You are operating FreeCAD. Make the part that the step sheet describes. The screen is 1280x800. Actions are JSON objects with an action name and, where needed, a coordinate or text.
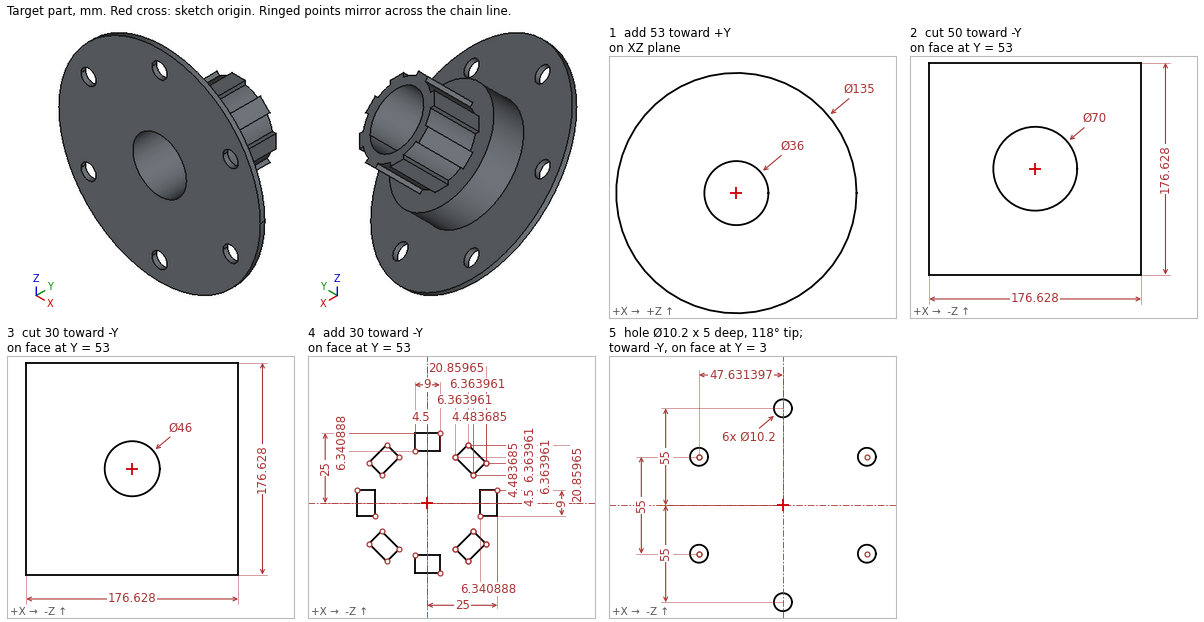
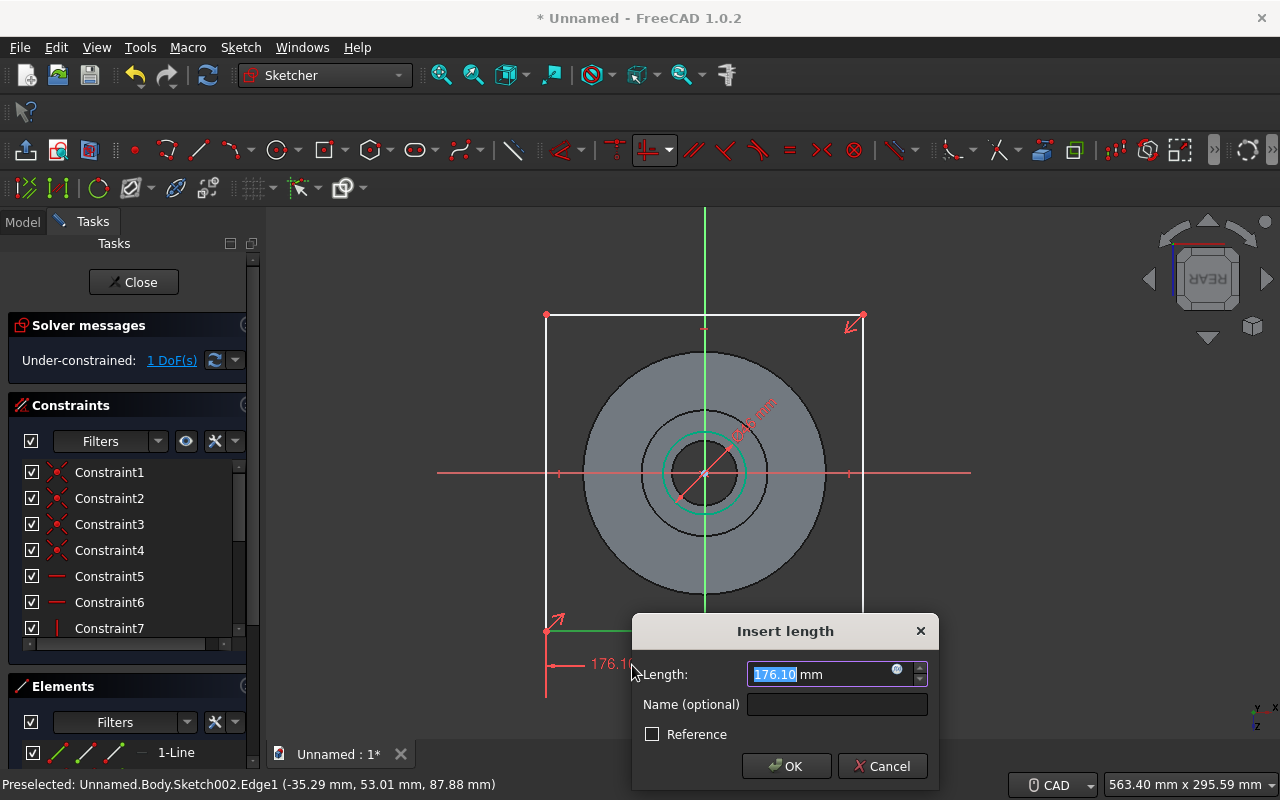
{"action": "type", "text": "176.628"}
{"action": "key", "text": "Return"}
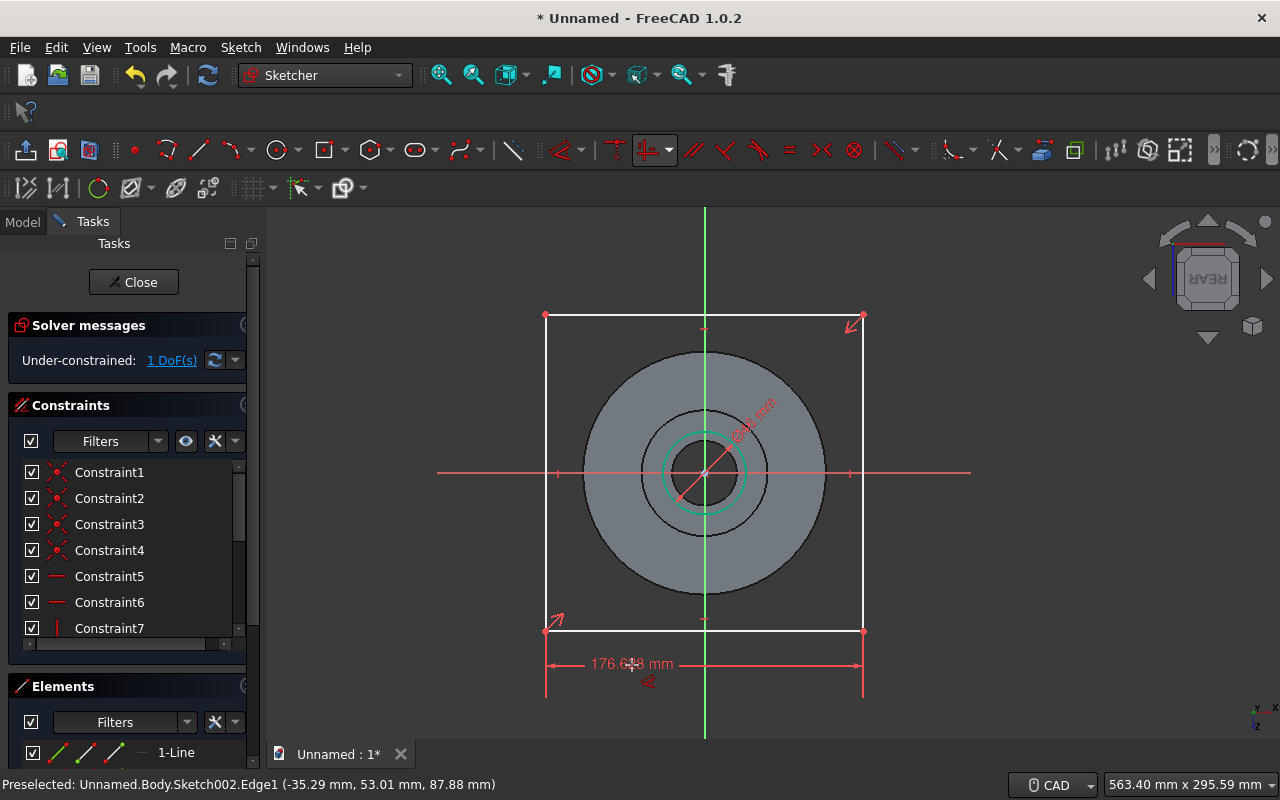
{"action": "left_click", "coordinate": [863, 536]}
{"action": "left_click", "coordinate": [897, 400]}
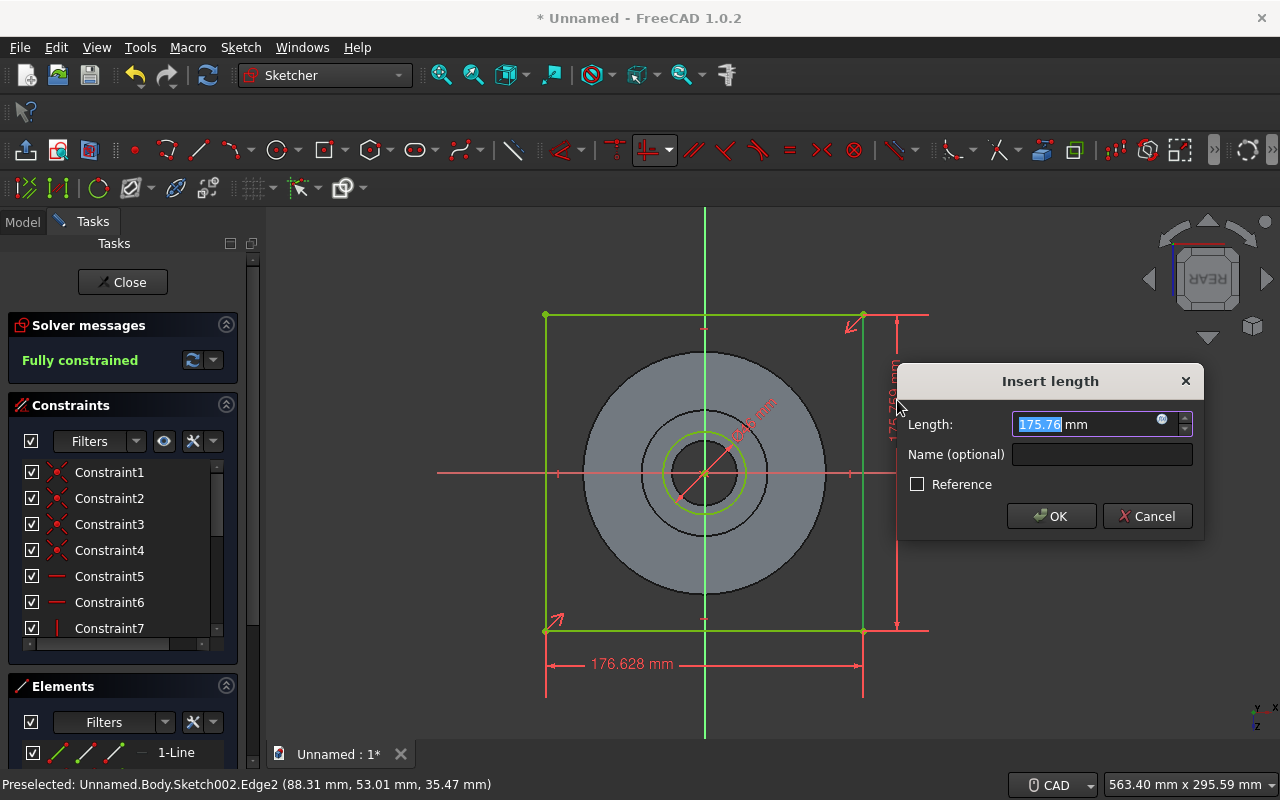
{"action": "type", "text": "176.628"}
{"action": "key", "text": "Return"}
{"action": "key", "text": "Escape"}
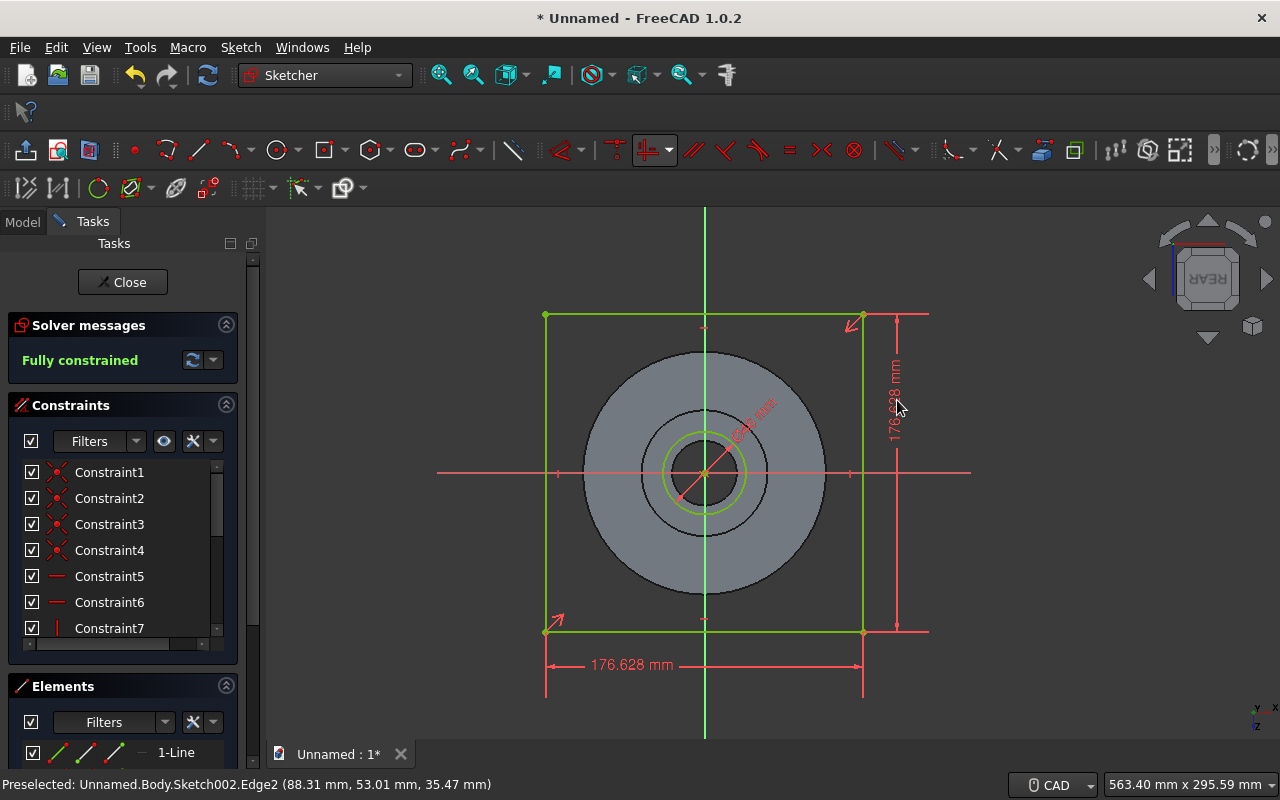
{"action": "left_click", "coordinate": [123, 282]}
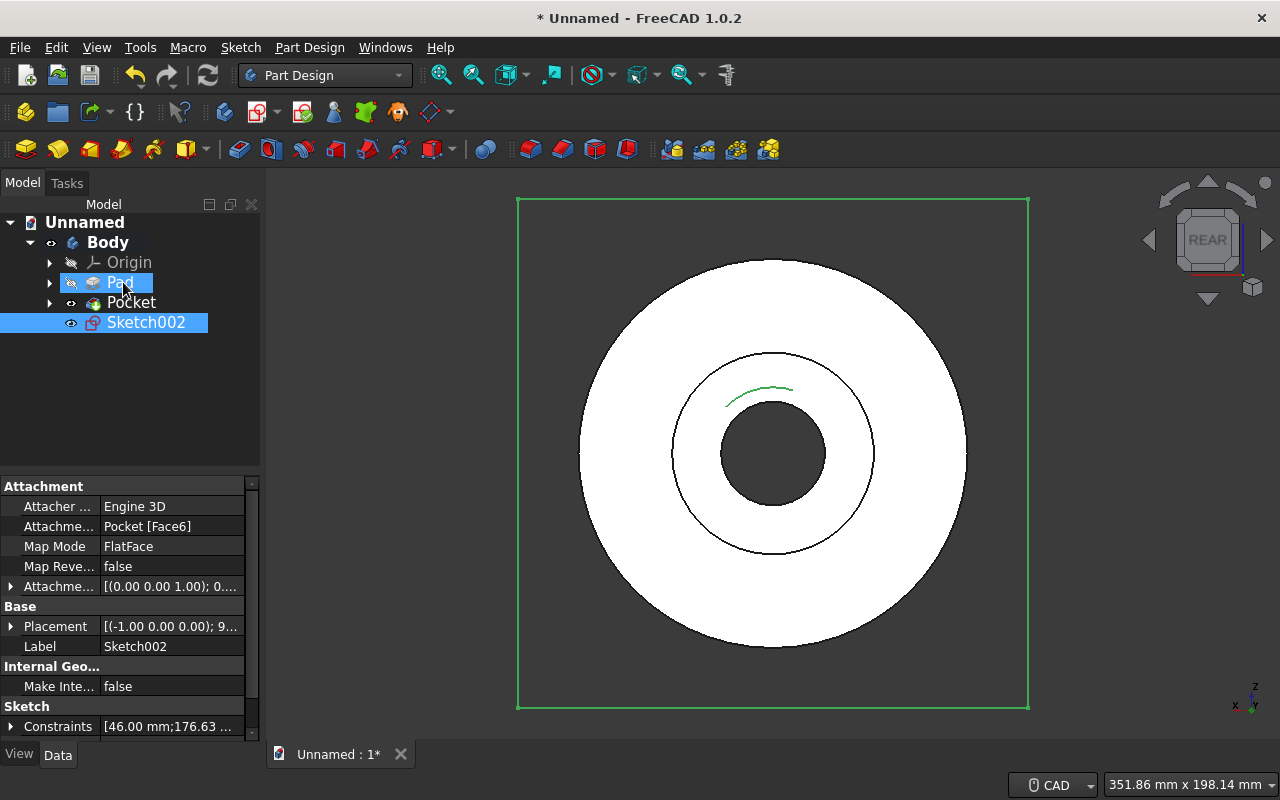
{"action": "left_click", "coordinate": [240, 150]}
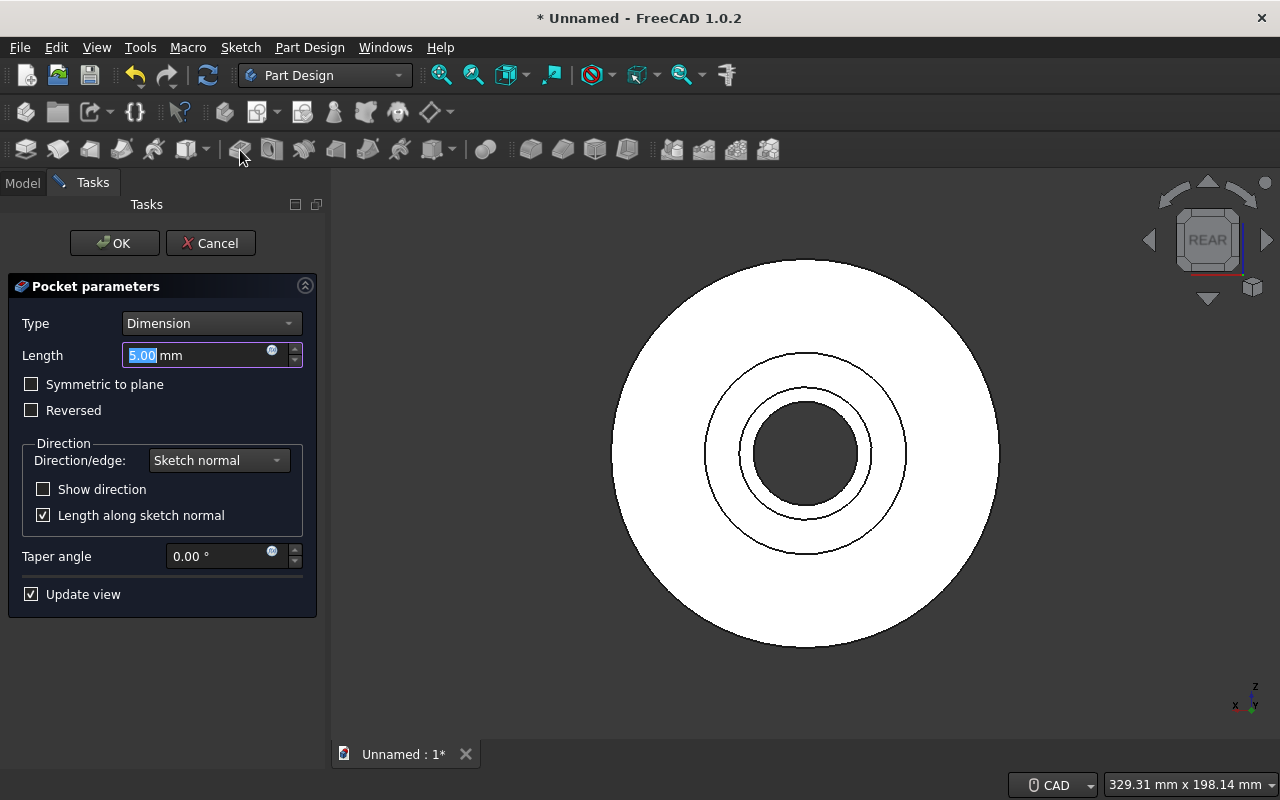
{"action": "type", "text": "30"}
{"action": "key", "text": "Tab"}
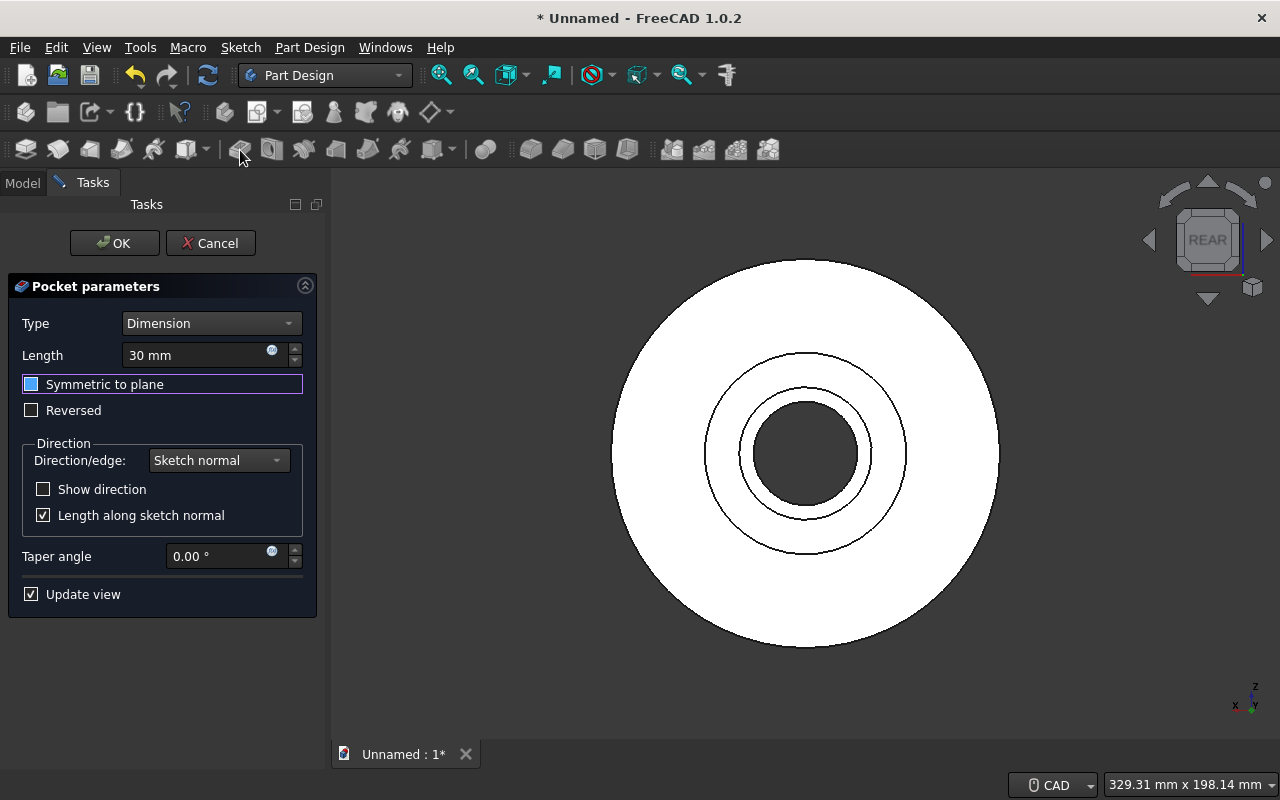
{"action": "left_click", "coordinate": [115, 243]}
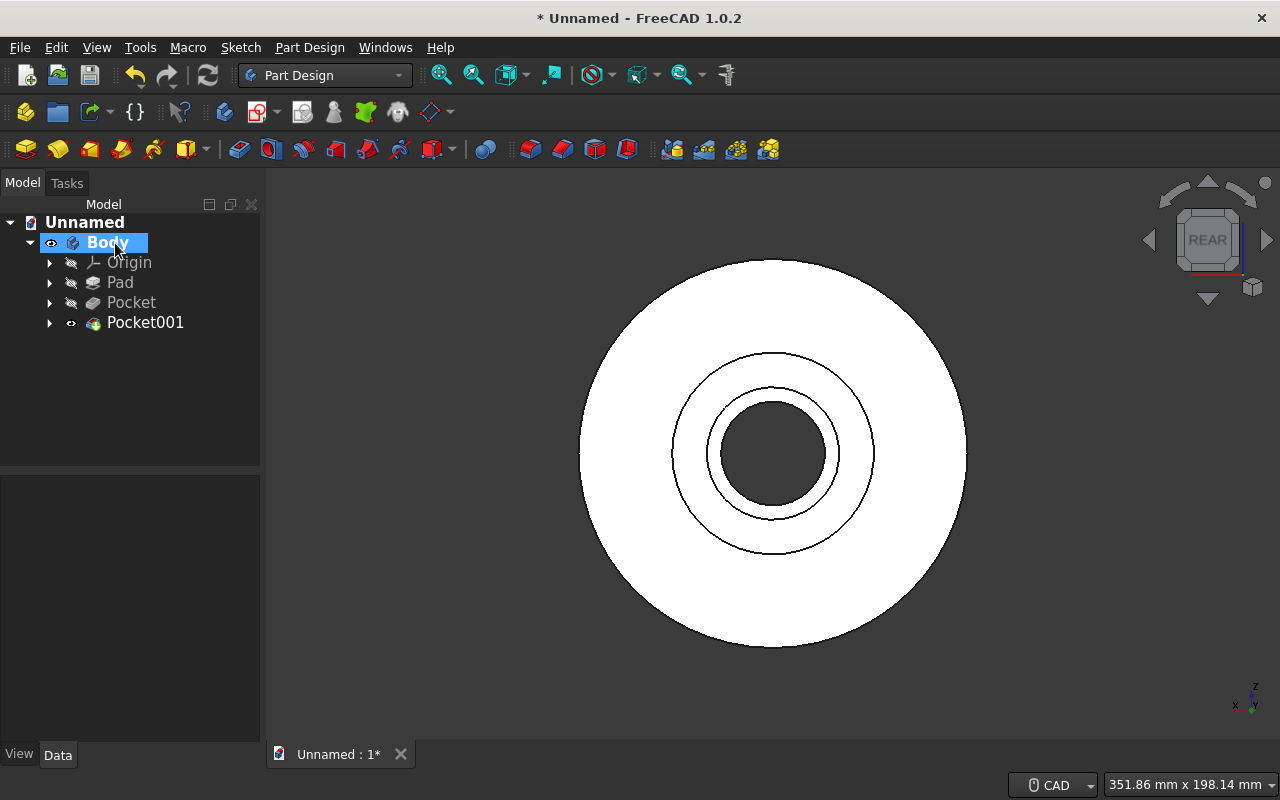
{"action": "scroll", "coordinate": [792, 509], "scroll_direction": "up", "scroll_amount": 4}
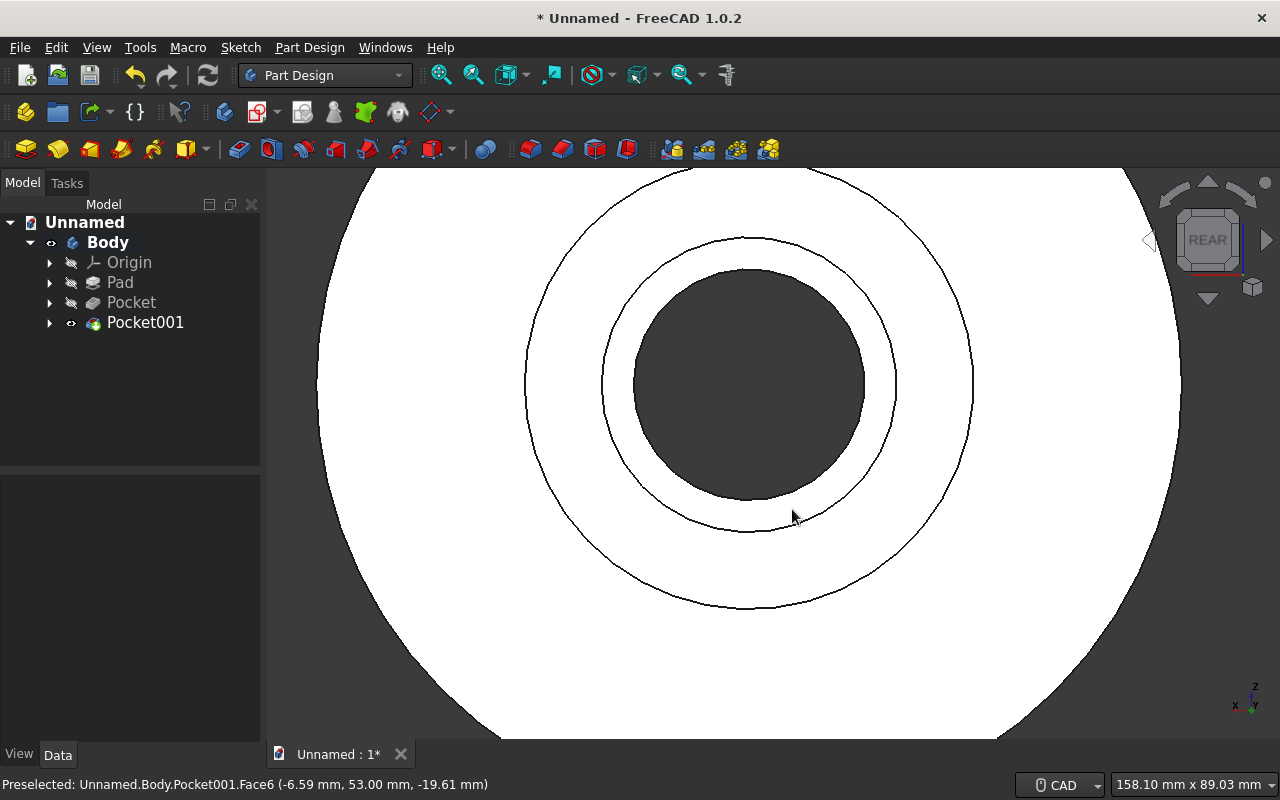
{"action": "left_click", "coordinate": [791, 510]}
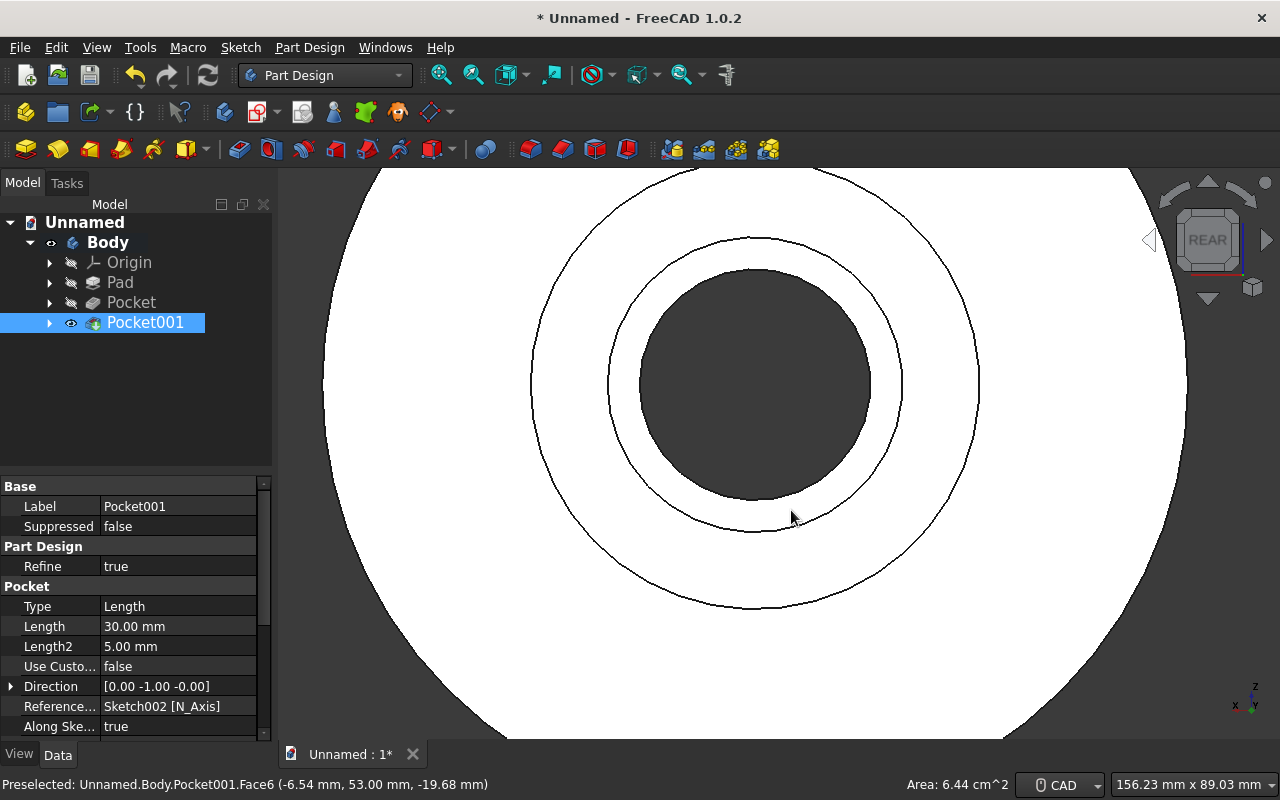
{"action": "left_click", "coordinate": [258, 112]}